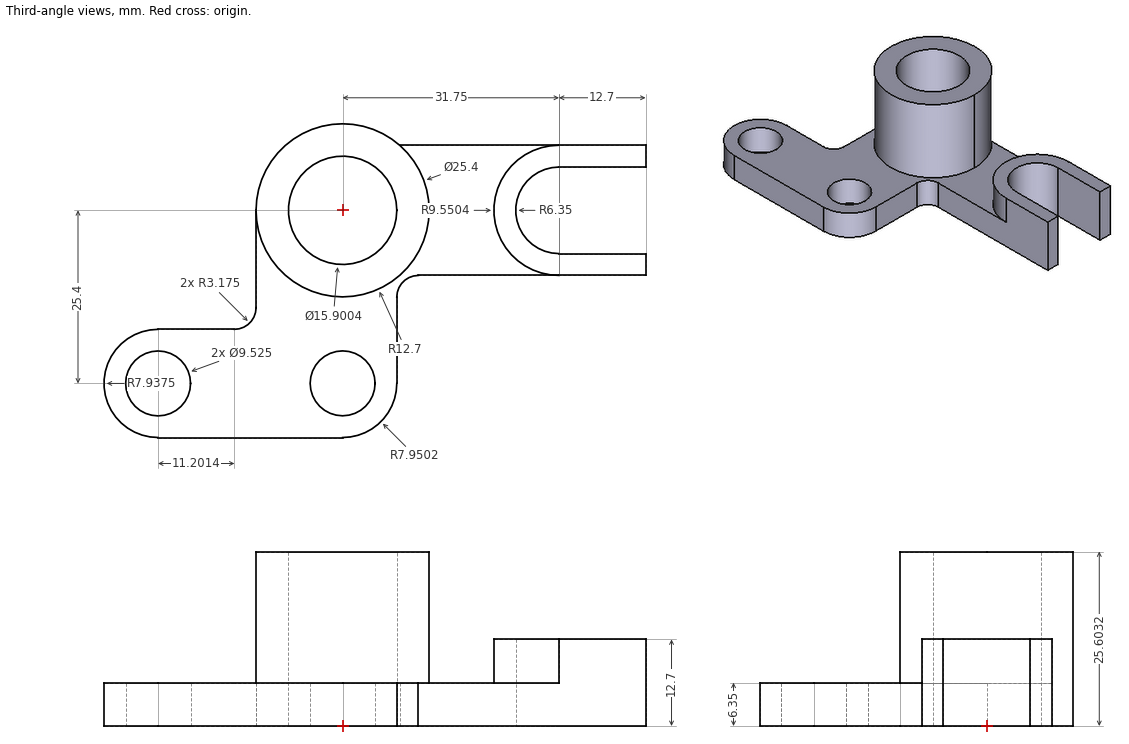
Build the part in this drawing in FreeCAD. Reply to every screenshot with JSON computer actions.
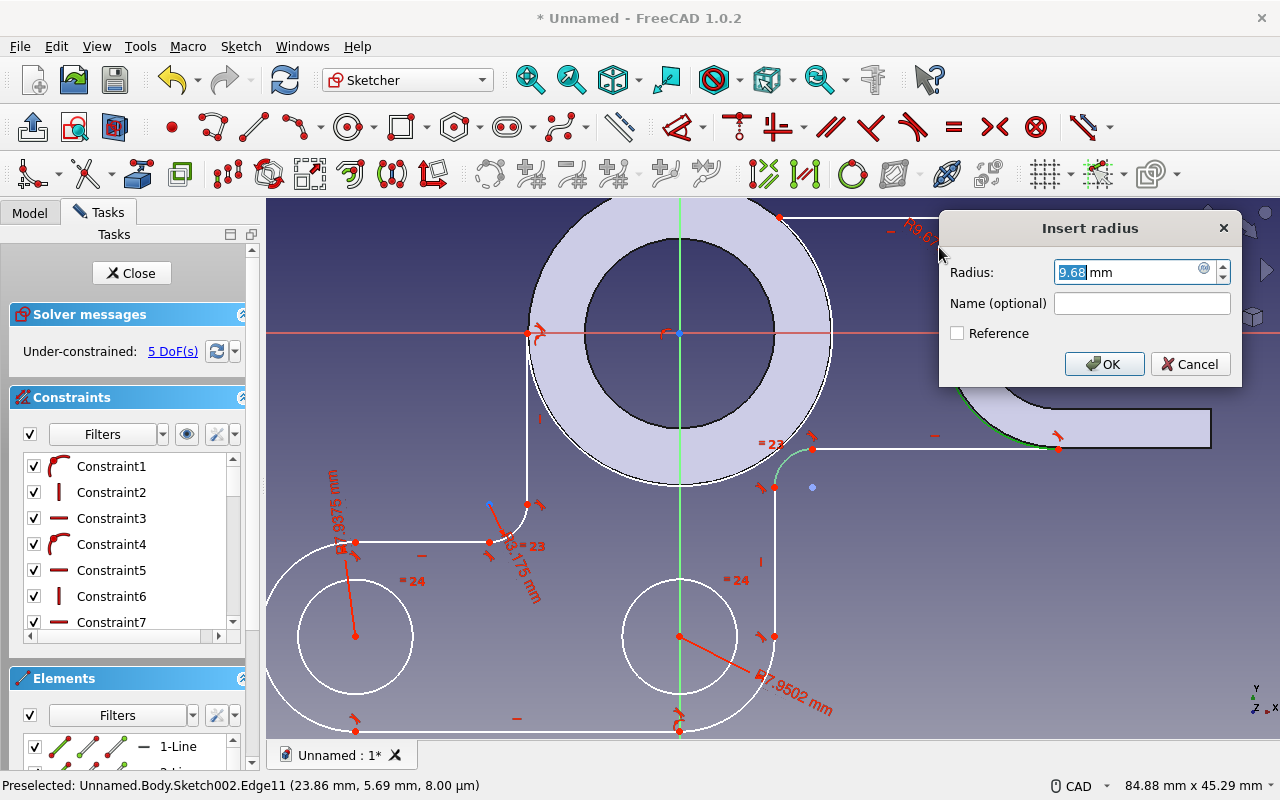
{"action": "type", "text": "9.5504"}
{"action": "key", "text": "Return"}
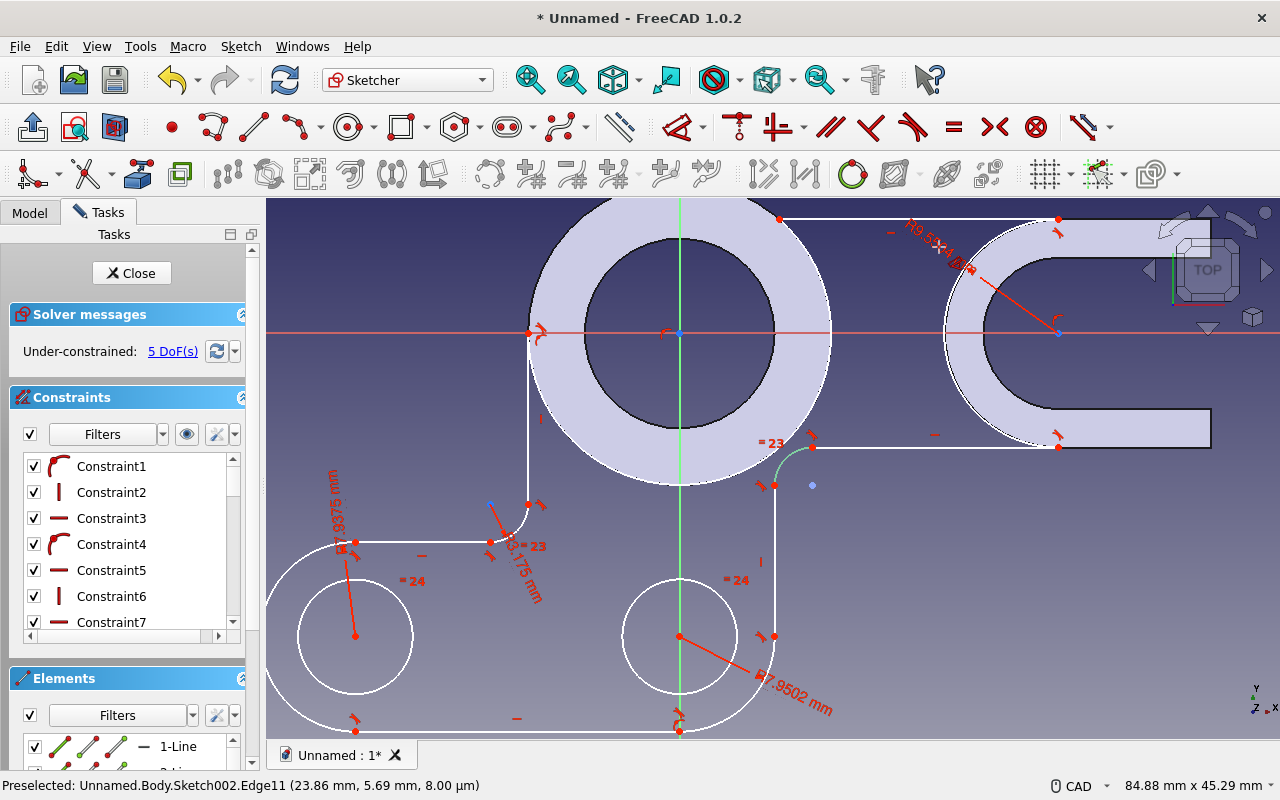
{"action": "left_click", "coordinate": [625, 475]}
{"action": "left_click", "coordinate": [613, 505]}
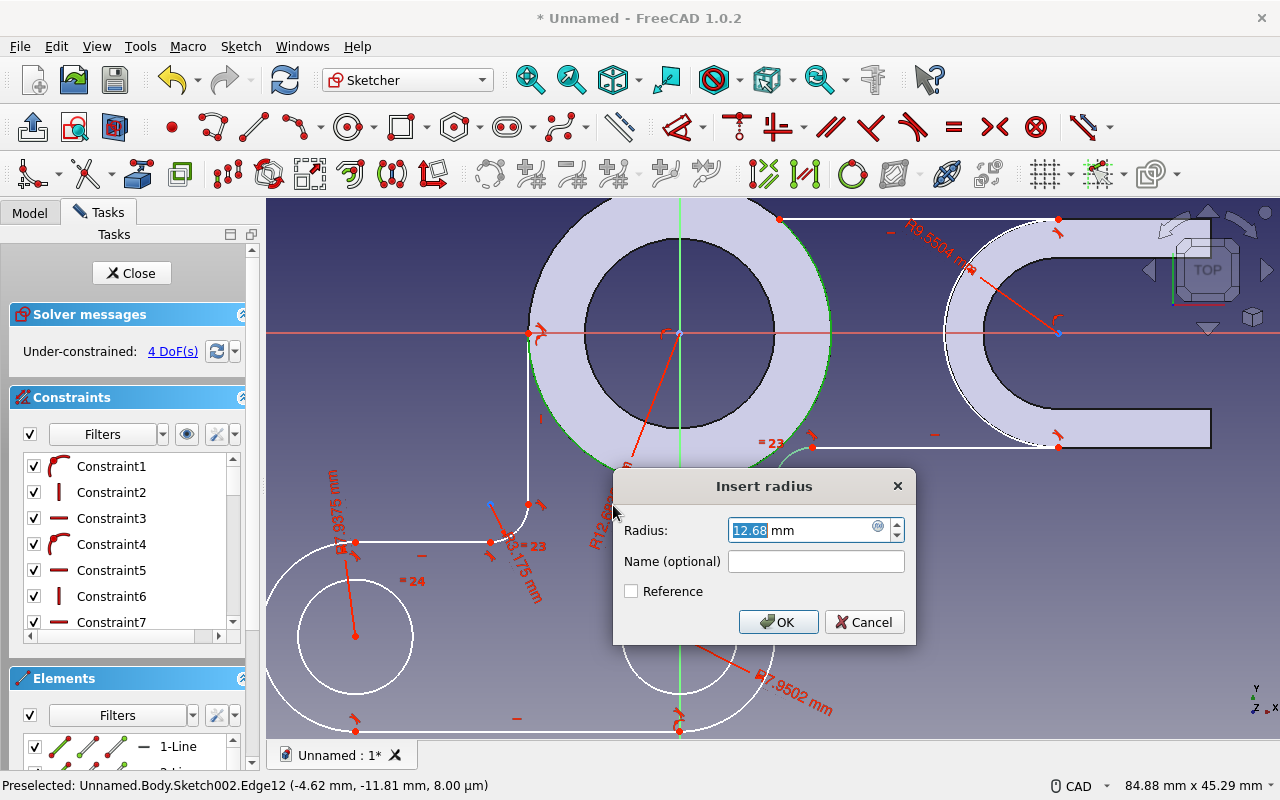
{"action": "type", "text": "12.7"}
{"action": "key", "text": "Return"}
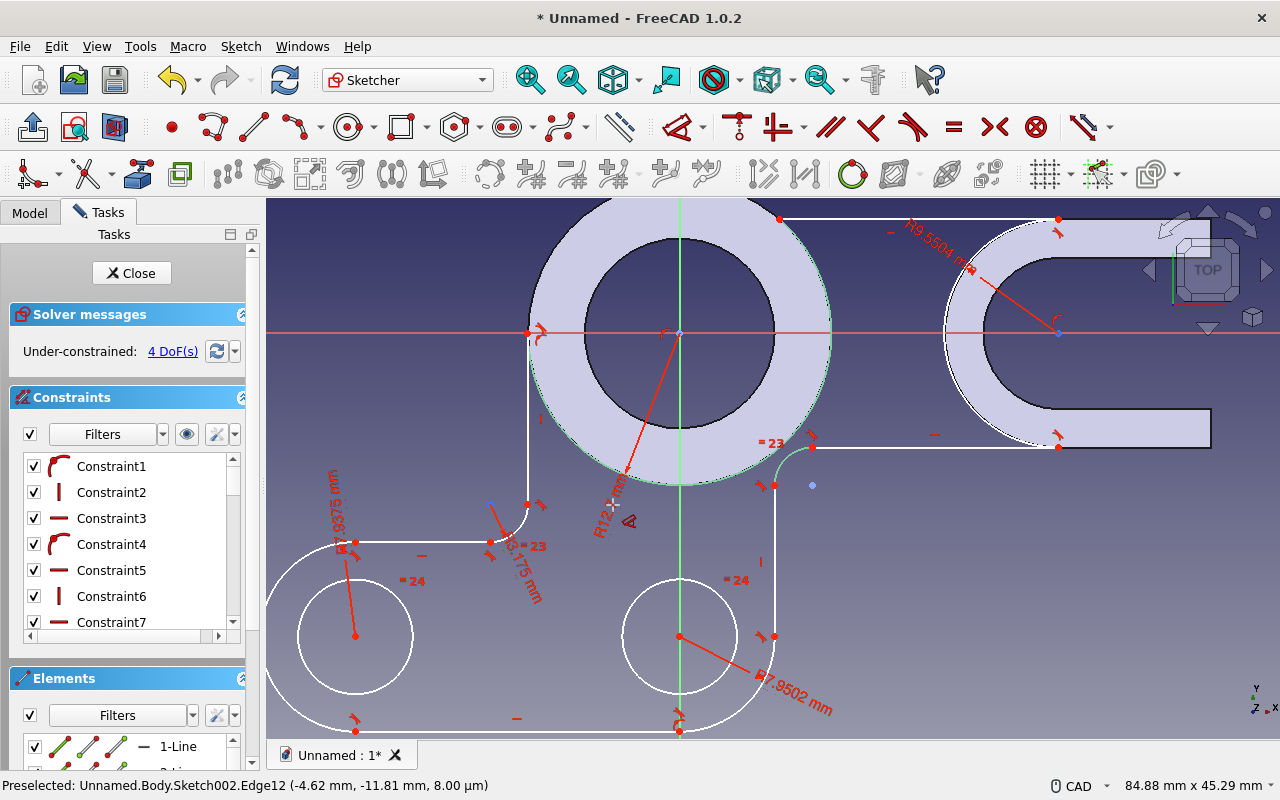
{"action": "left_click", "coordinate": [396, 596]}
{"action": "left_click", "coordinate": [419, 573]}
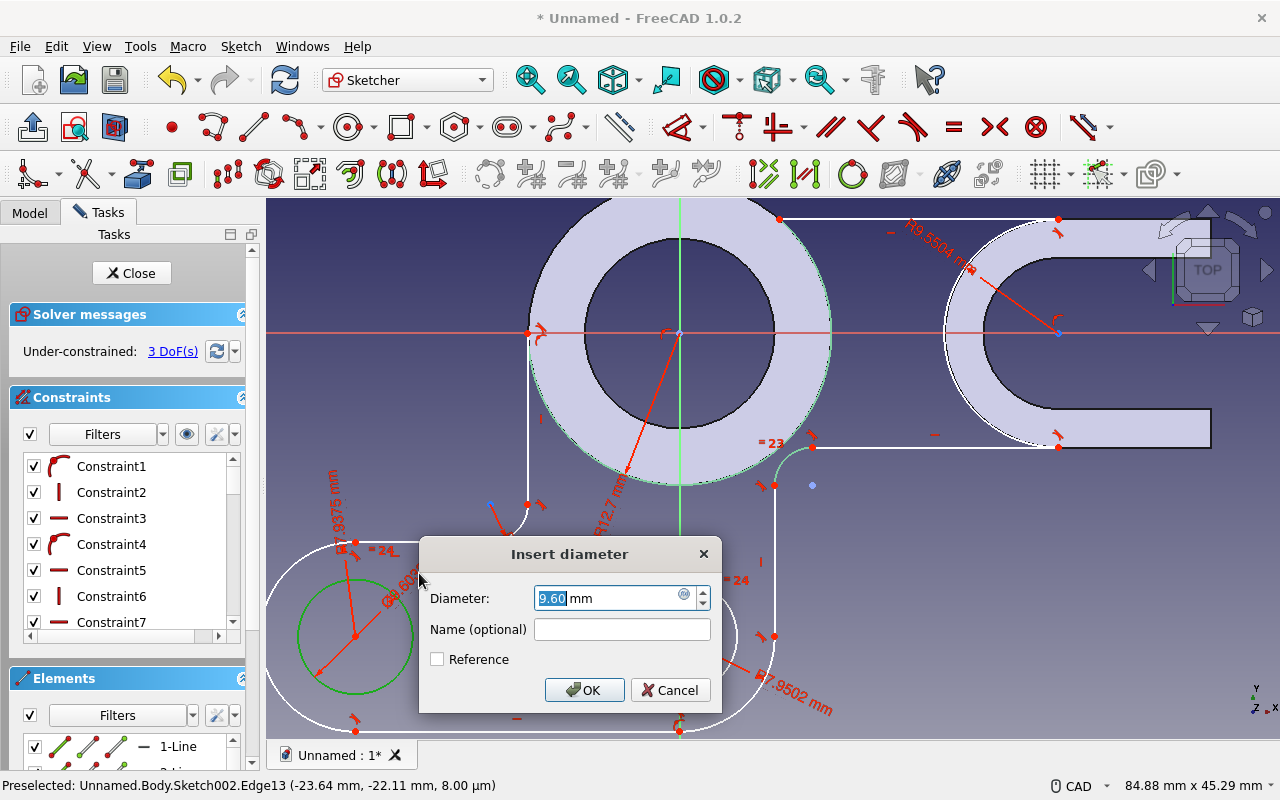
{"action": "type", "text": "9.525"}
{"action": "key", "text": "Return"}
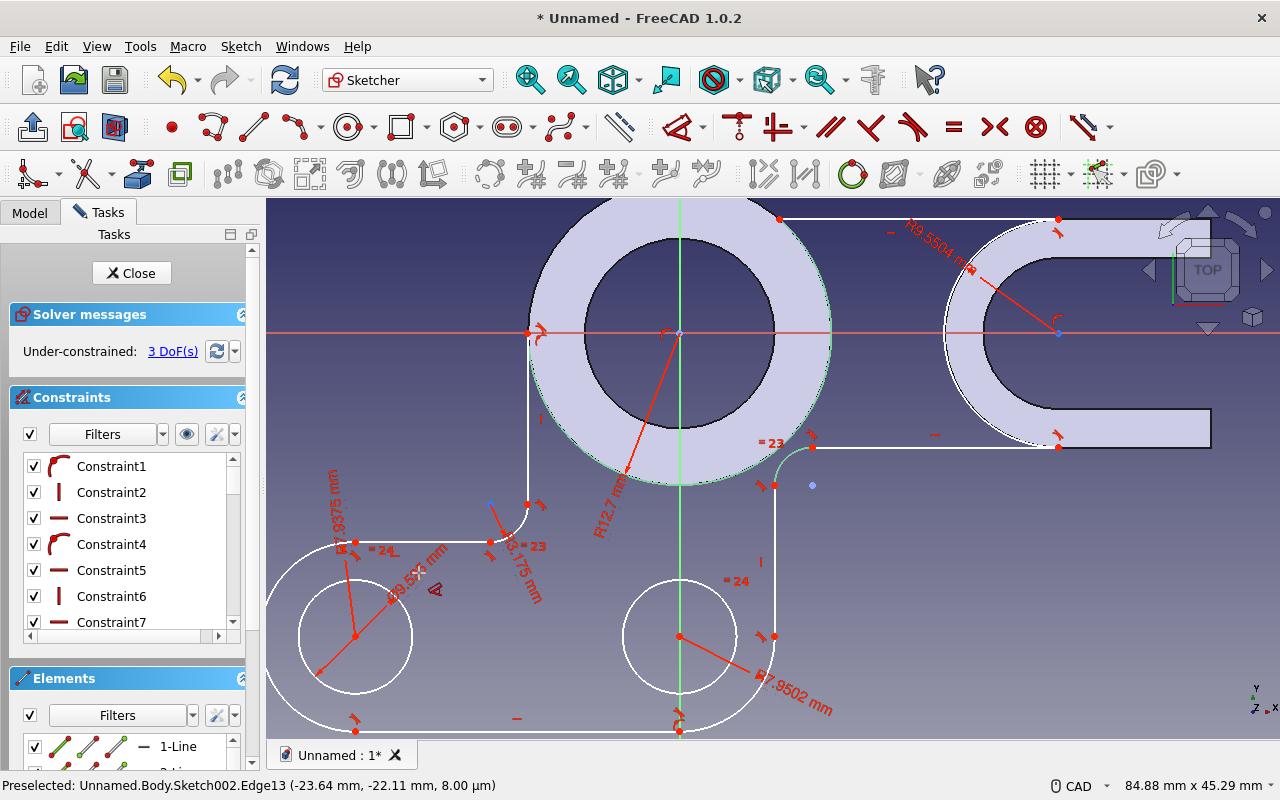
{"action": "left_click", "coordinate": [355, 637]}
{"action": "left_click", "coordinate": [321, 485]}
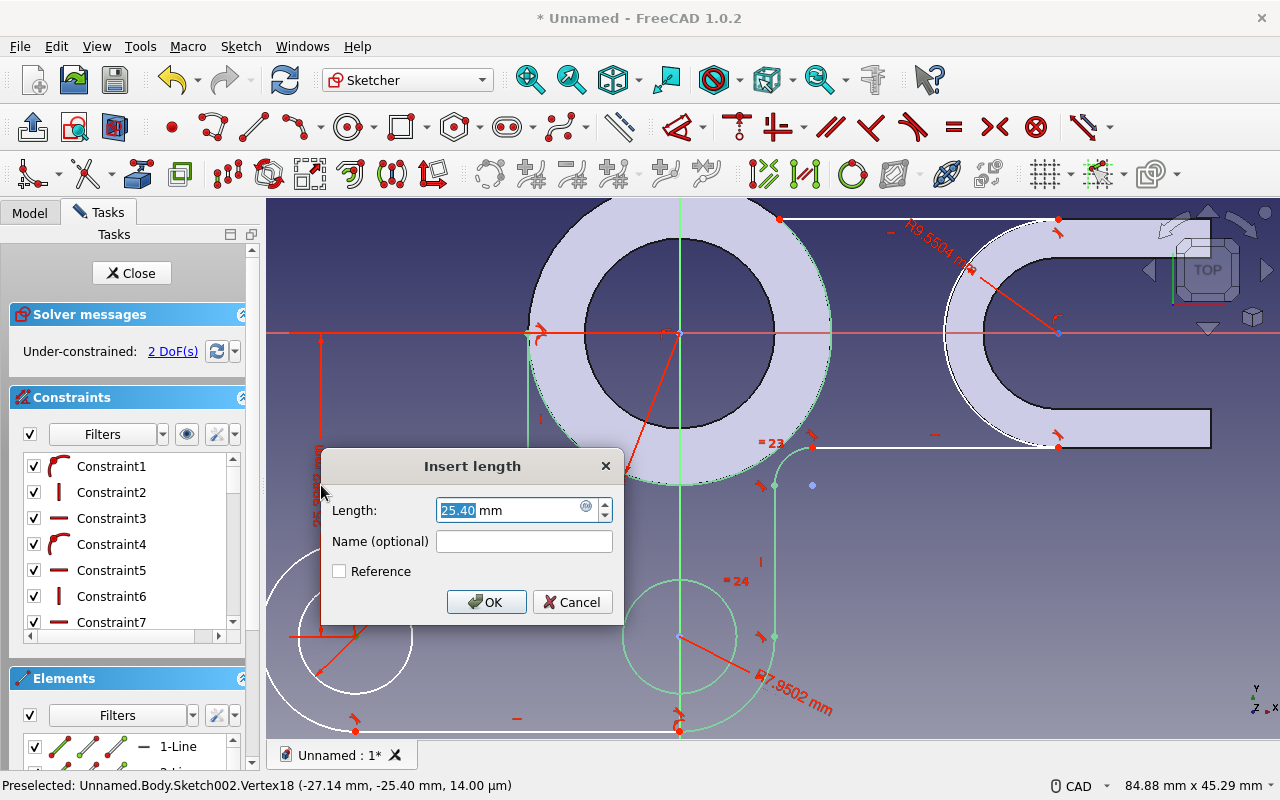
{"action": "type", "text": "25.4"}
{"action": "key", "text": "Return"}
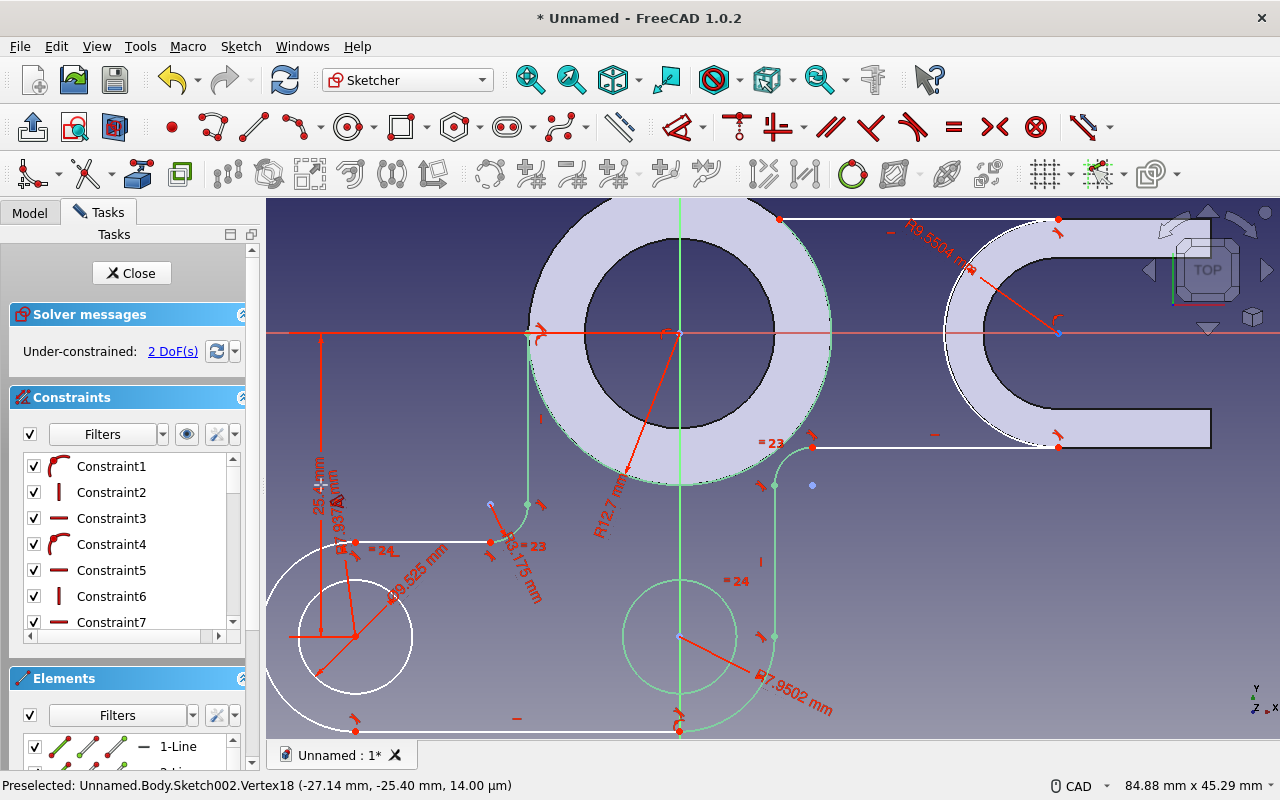
{"action": "left_click", "coordinate": [1058, 448]}
{"action": "left_click", "coordinate": [869, 299]}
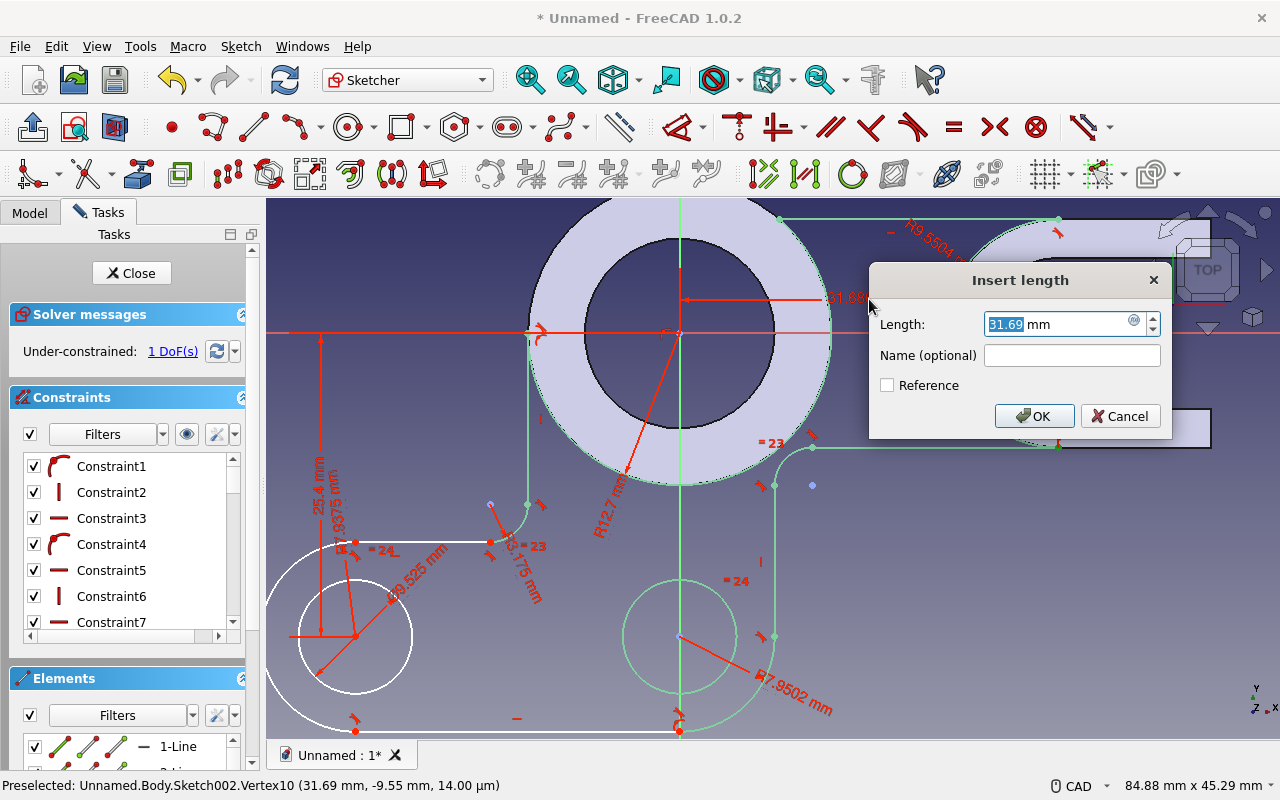
{"action": "type", "text": "31.75"}
{"action": "key", "text": "Return"}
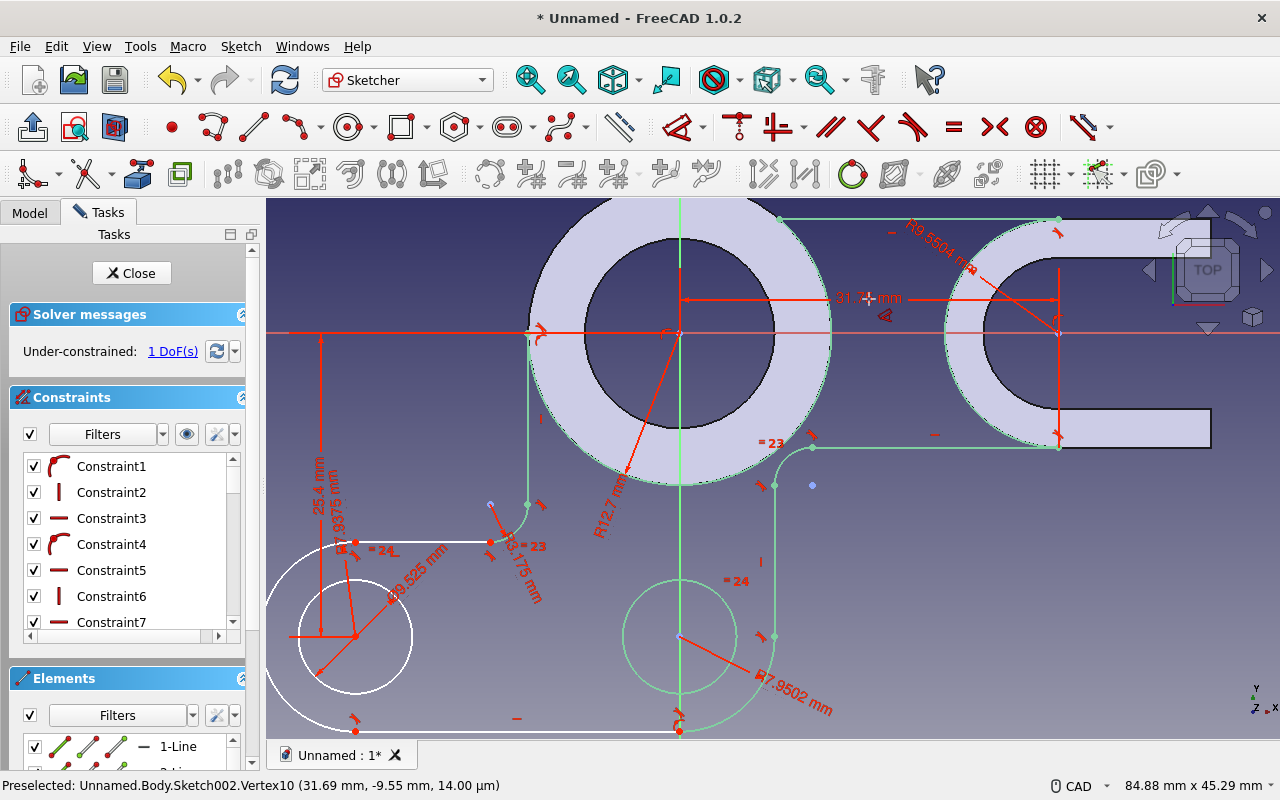
{"action": "left_click", "coordinate": [450, 542]}
{"action": "left_click", "coordinate": [423, 508]}